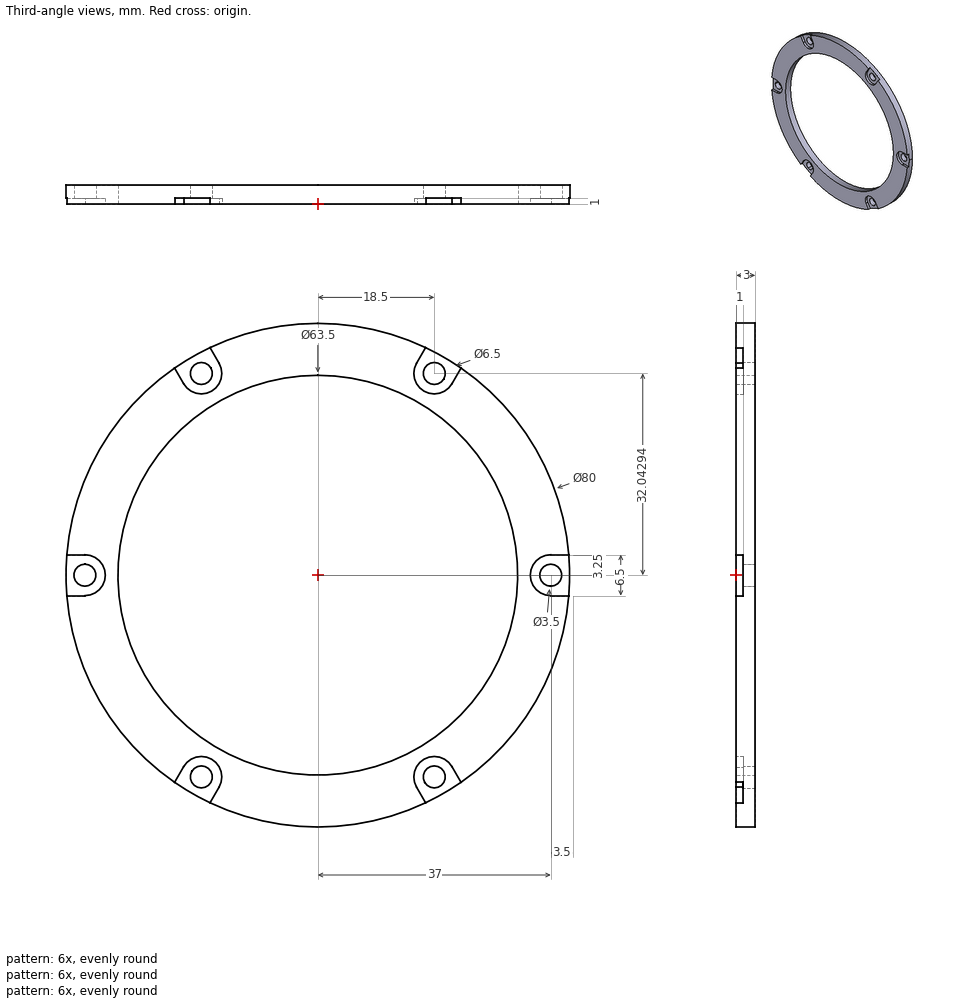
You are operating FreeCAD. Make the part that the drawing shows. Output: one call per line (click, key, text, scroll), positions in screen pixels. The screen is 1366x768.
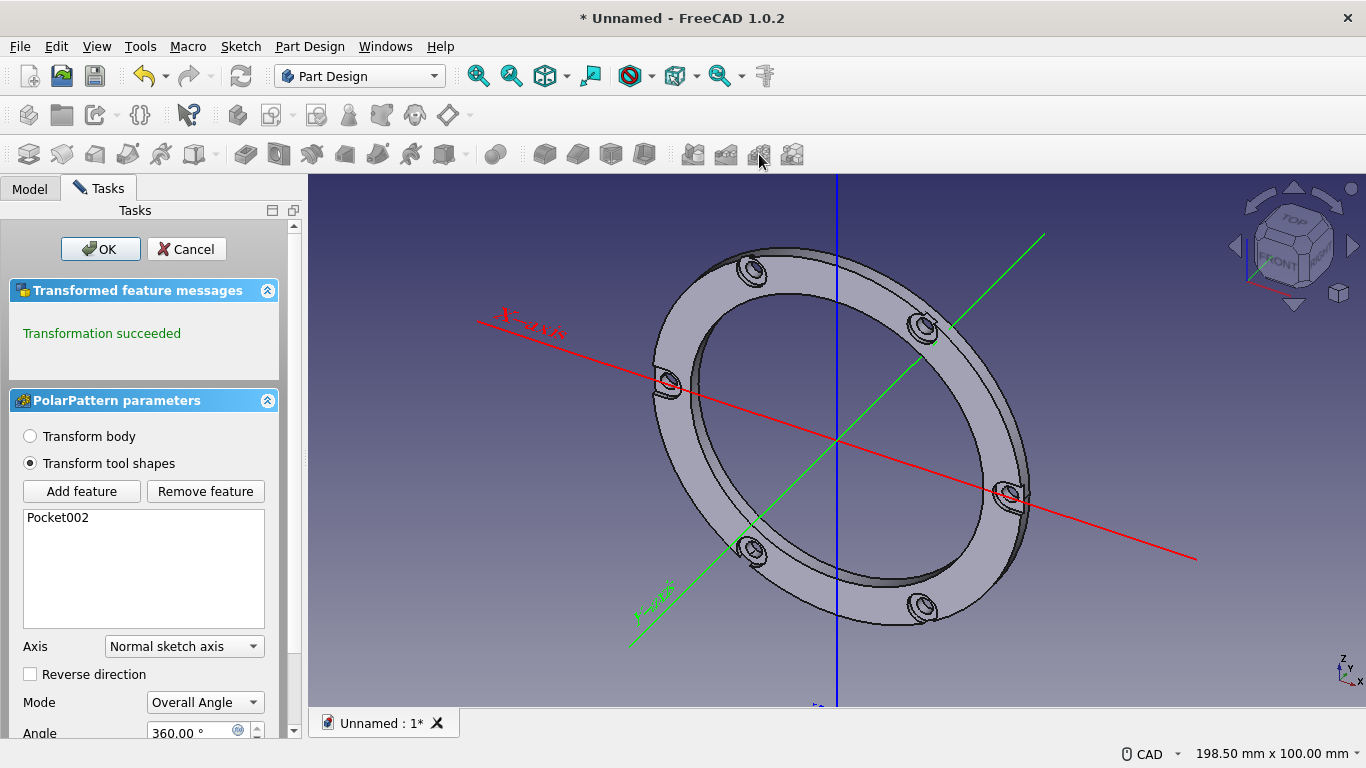
click(185, 646)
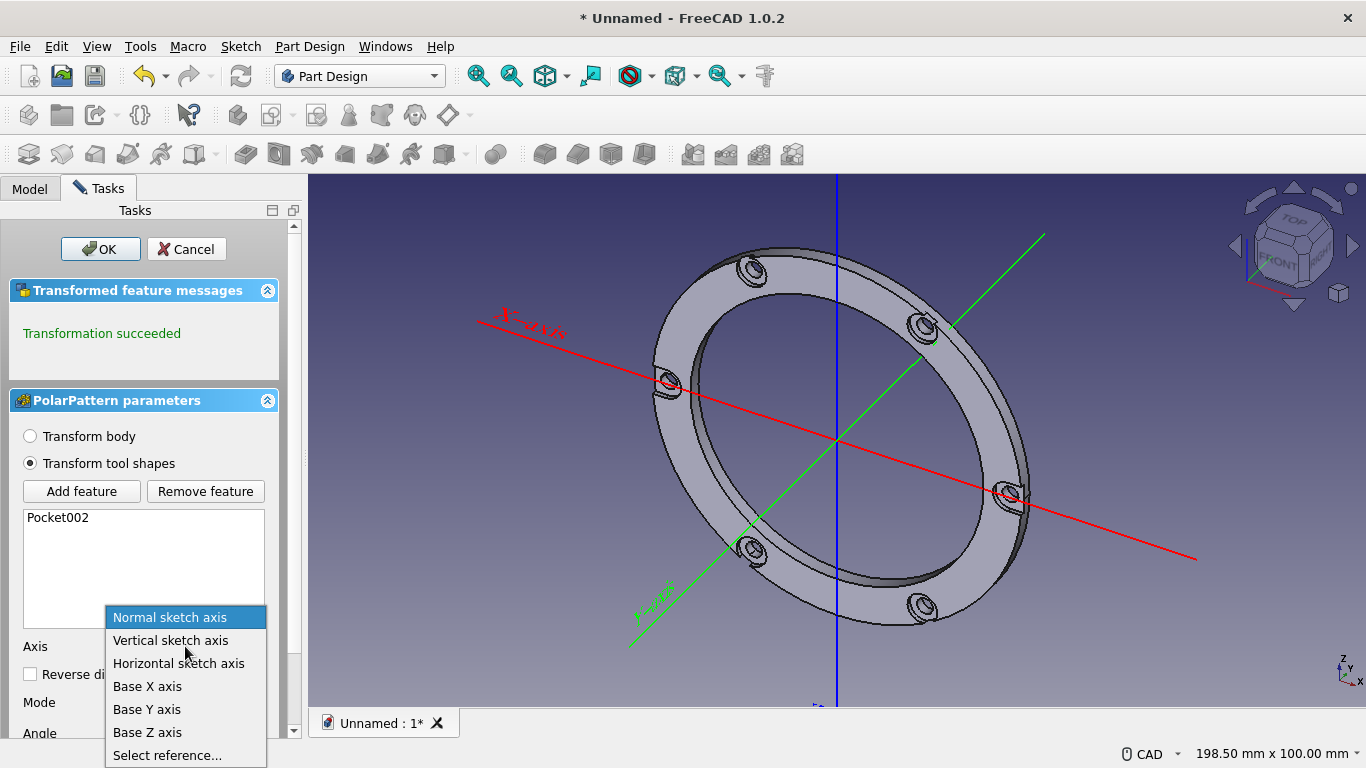
click(184, 710)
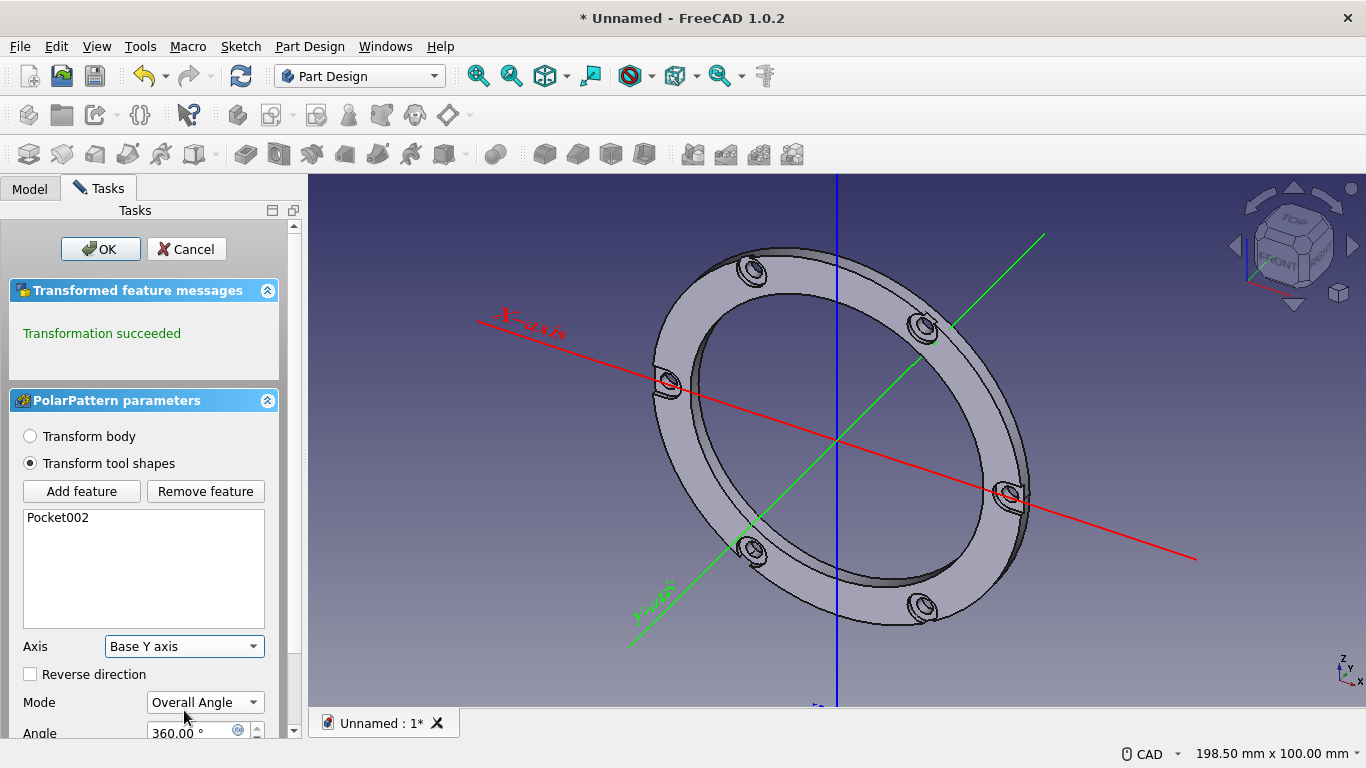
scroll(294, 479, down, 2)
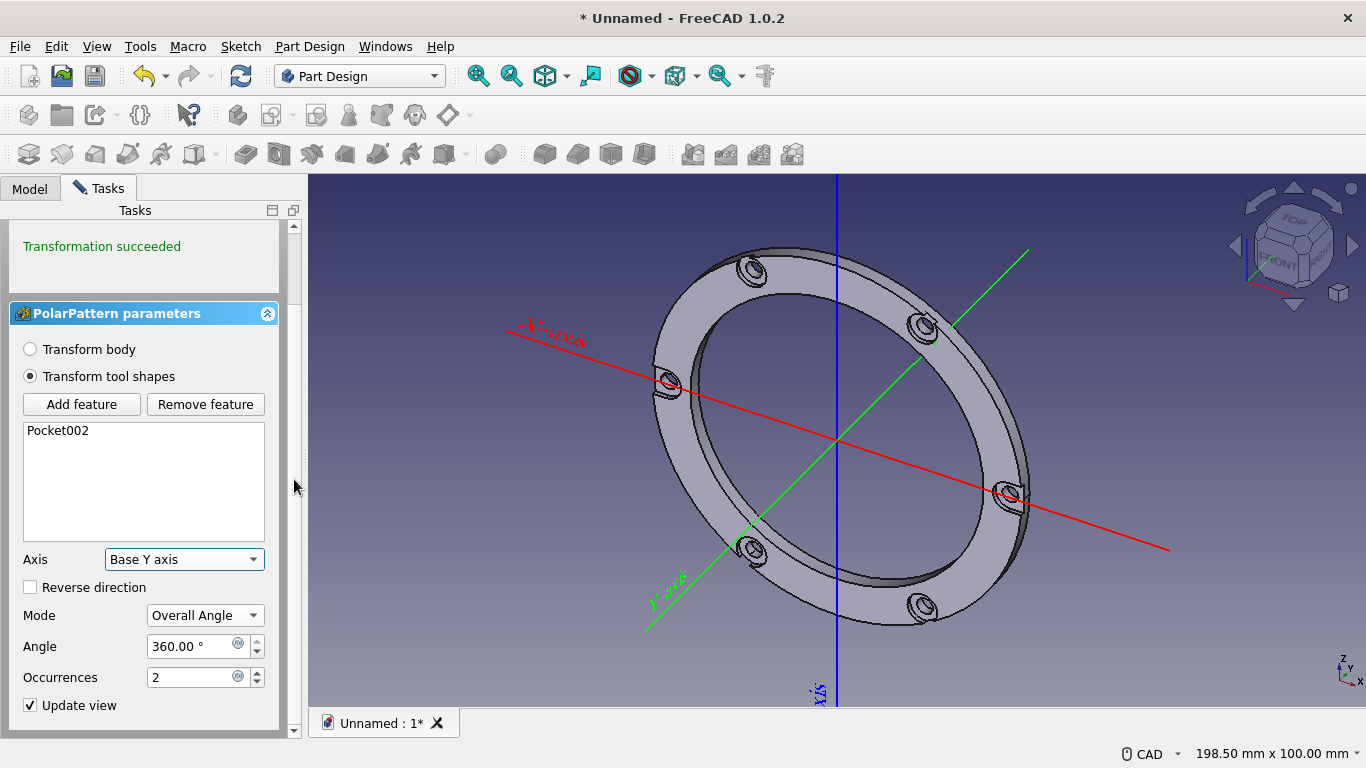
triple_click(199, 678)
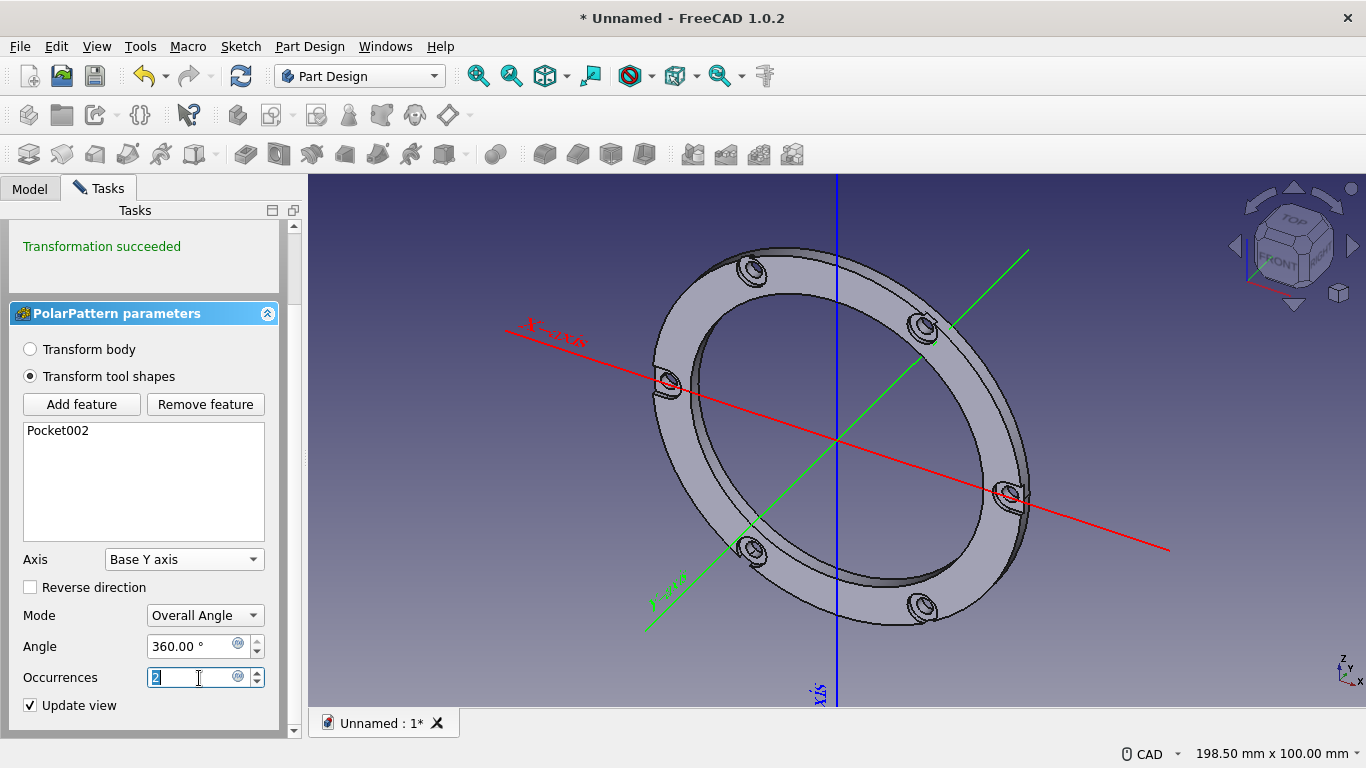
text(6)
key(Tab)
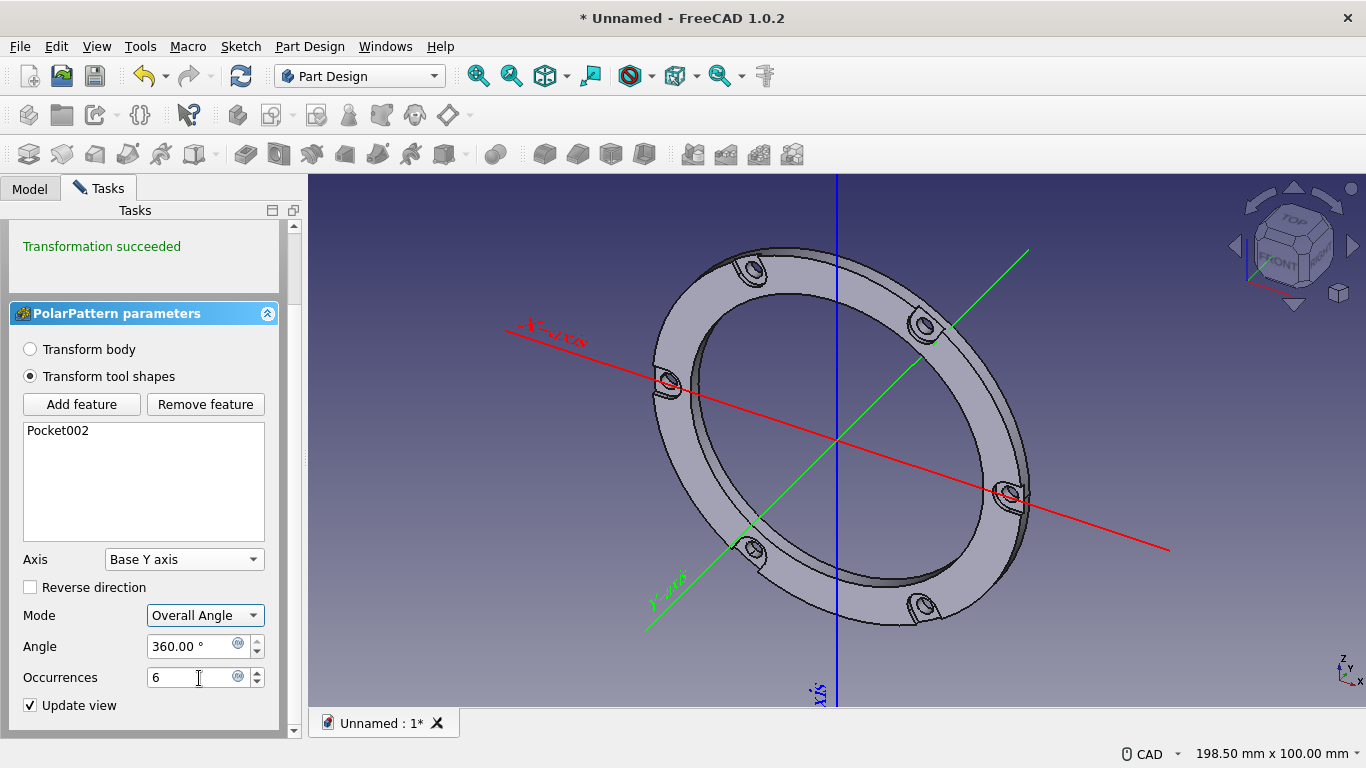
scroll(294, 479, up, 3)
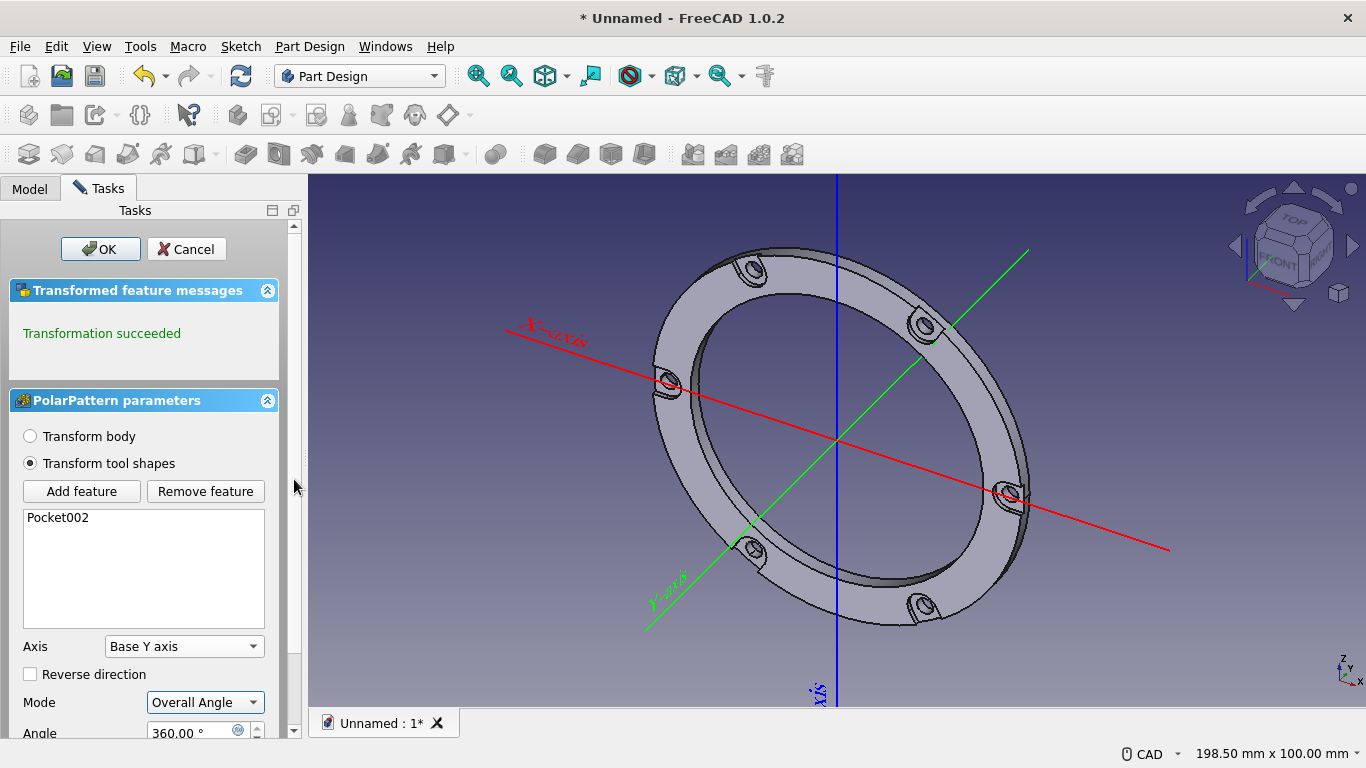
click(101, 249)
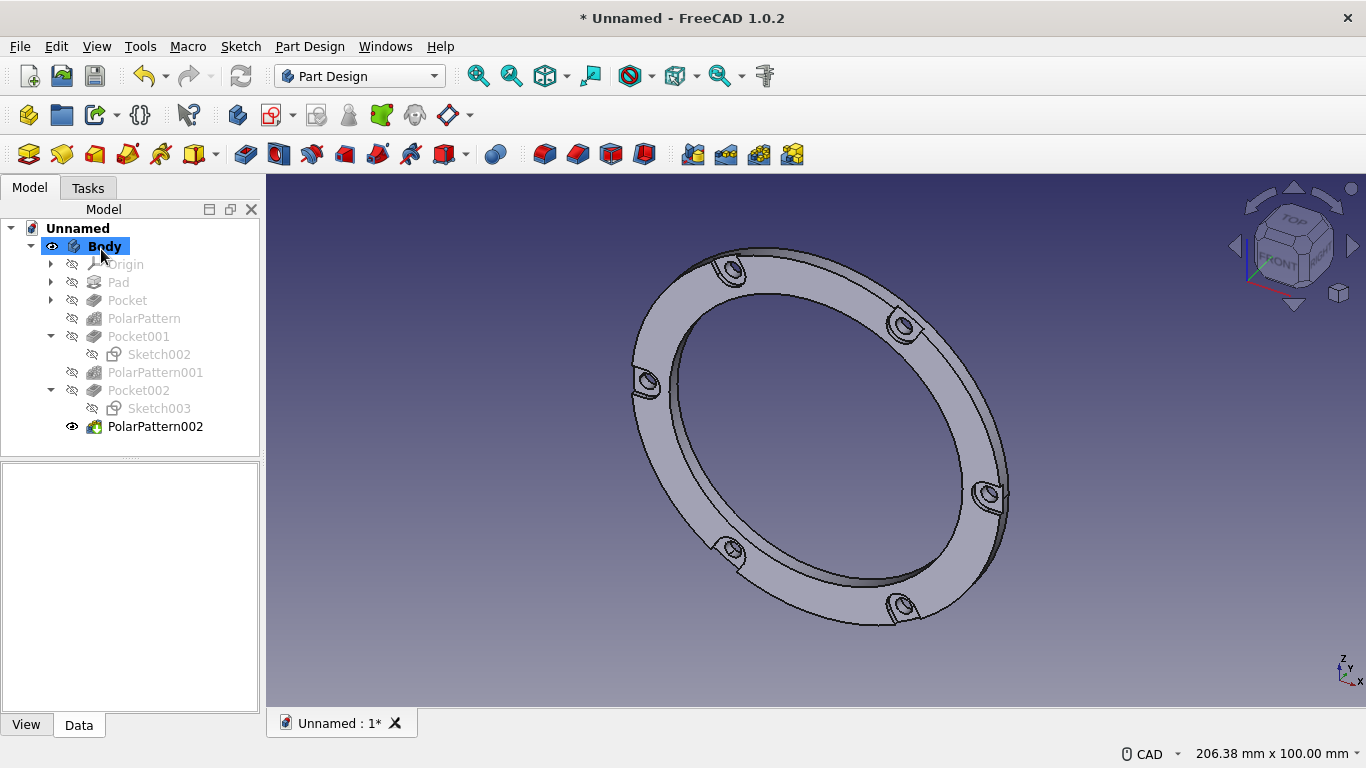
key(0)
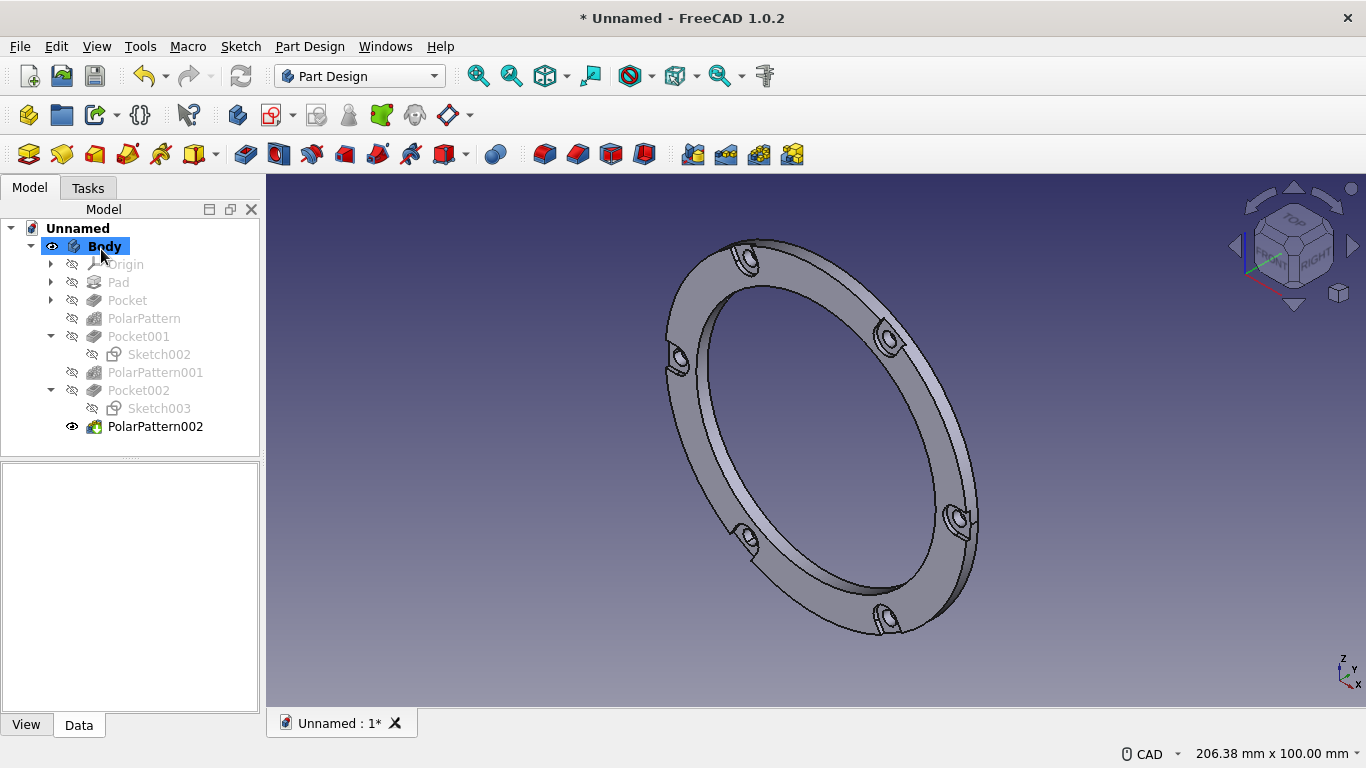
click(479, 76)